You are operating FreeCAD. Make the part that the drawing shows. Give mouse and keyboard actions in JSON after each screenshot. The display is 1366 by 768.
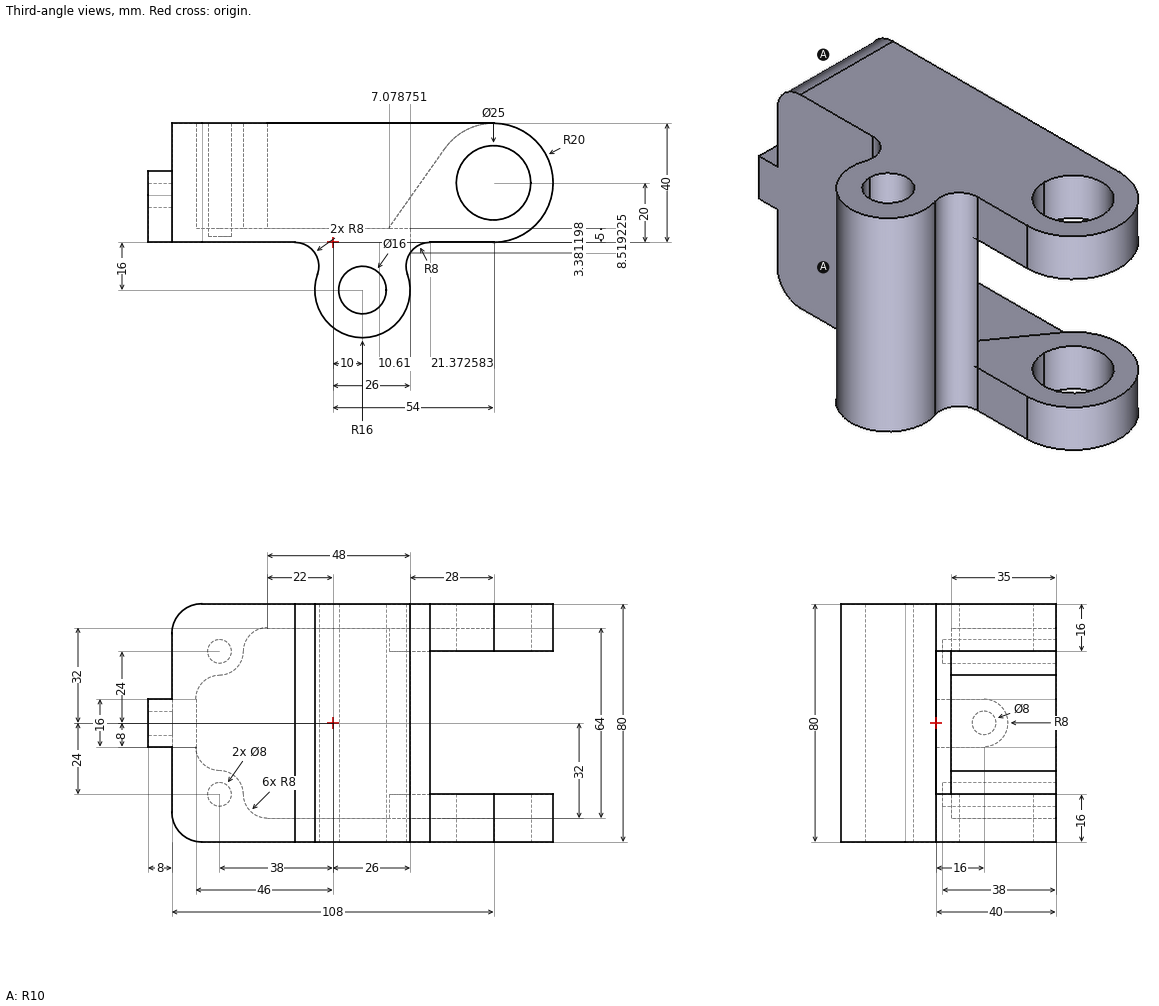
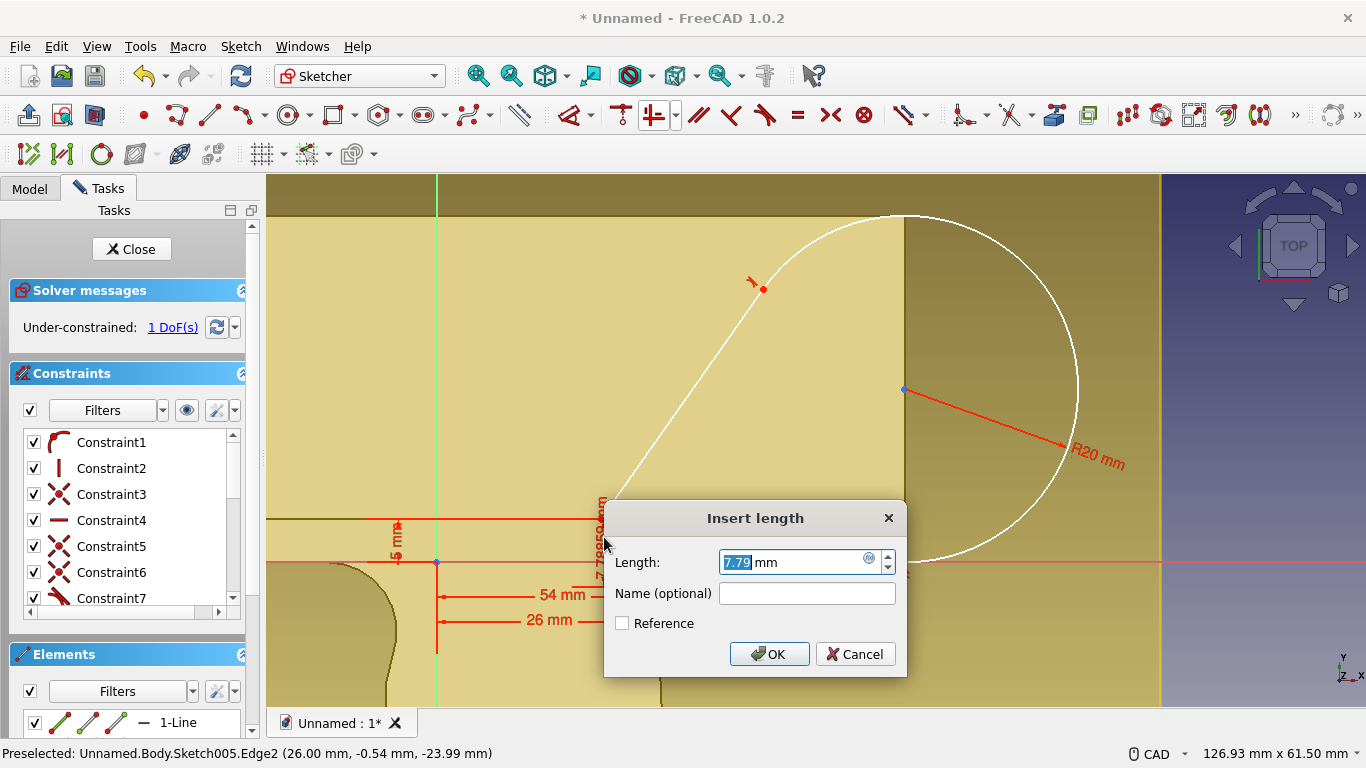
{"action": "type", "text": "8.519225"}
{"action": "key", "text": "Return"}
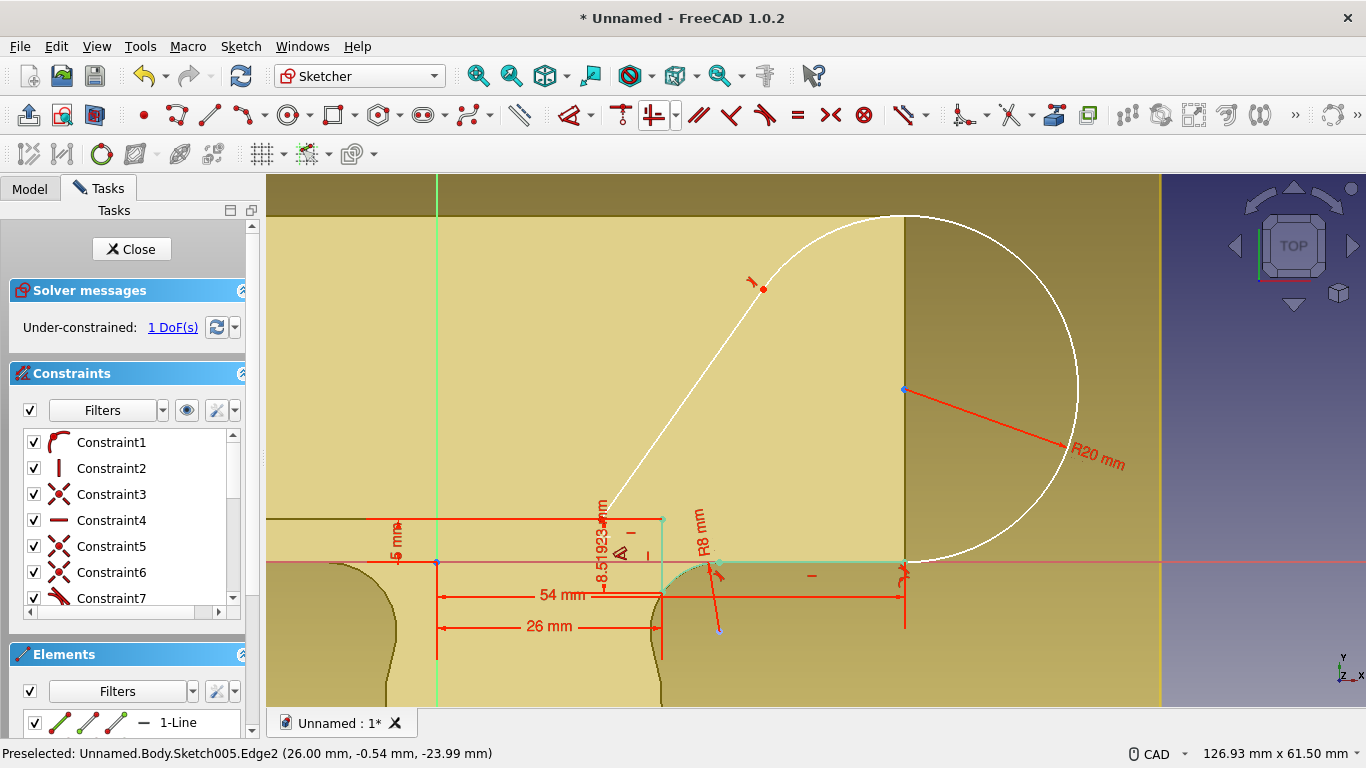
{"action": "left_click", "coordinate": [644, 519]}
{"action": "left_click", "coordinate": [646, 485]}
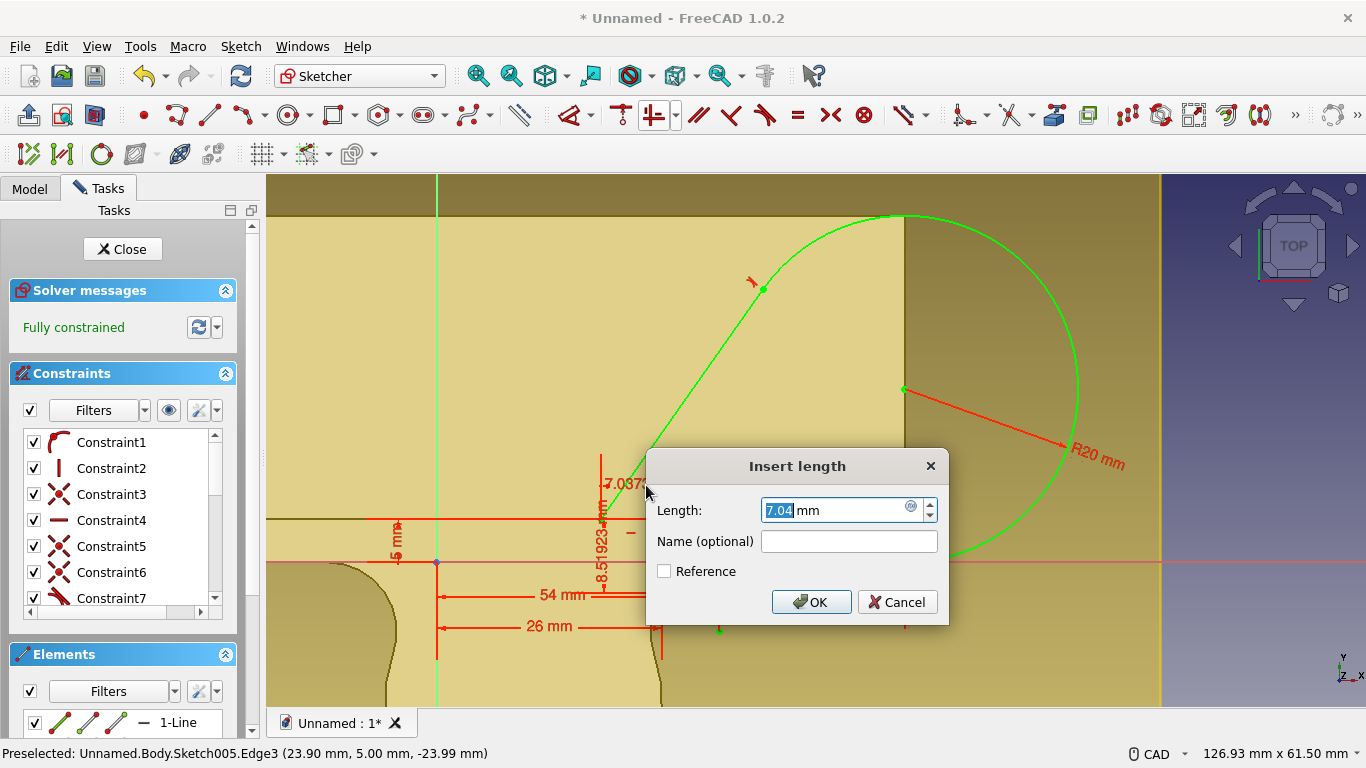
{"action": "type", "text": "7.078751"}
{"action": "key", "text": "Return"}
{"action": "key", "text": "Escape"}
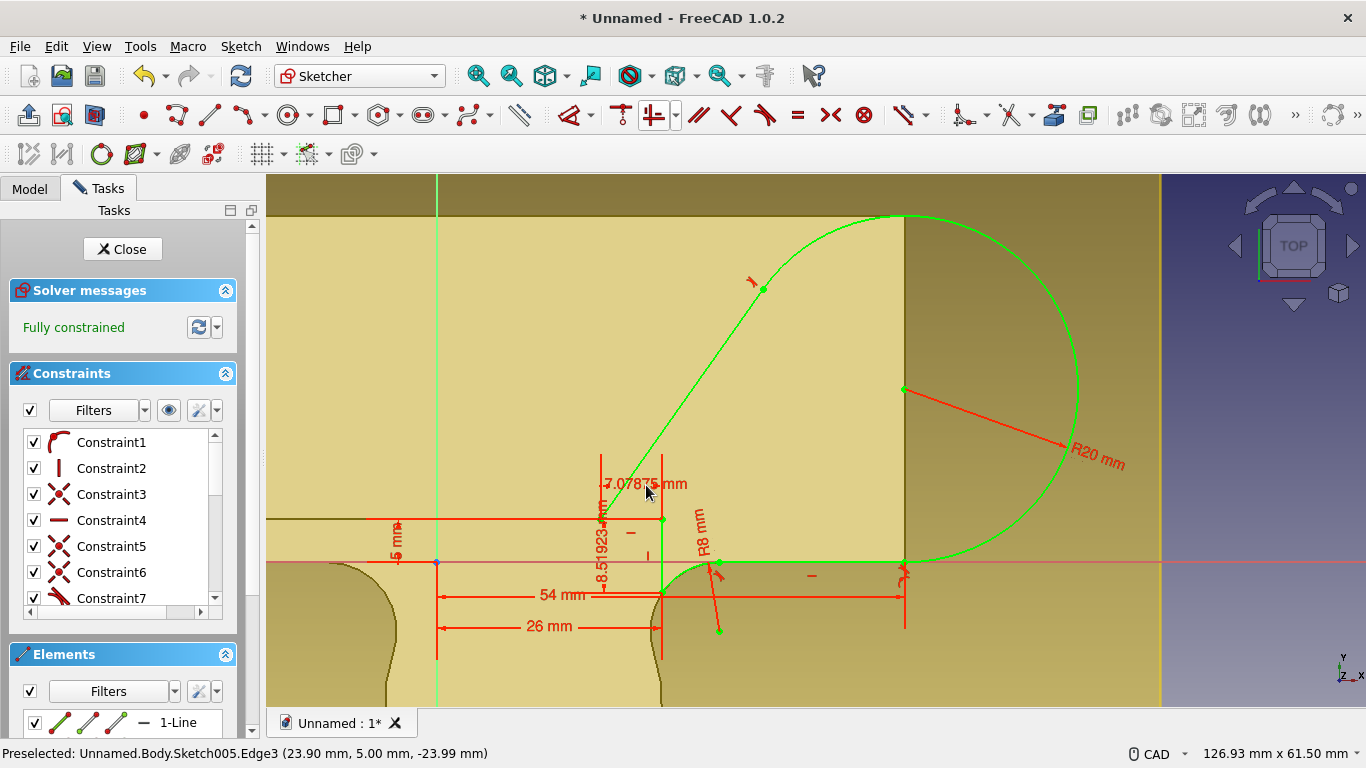
{"action": "left_click", "coordinate": [123, 249]}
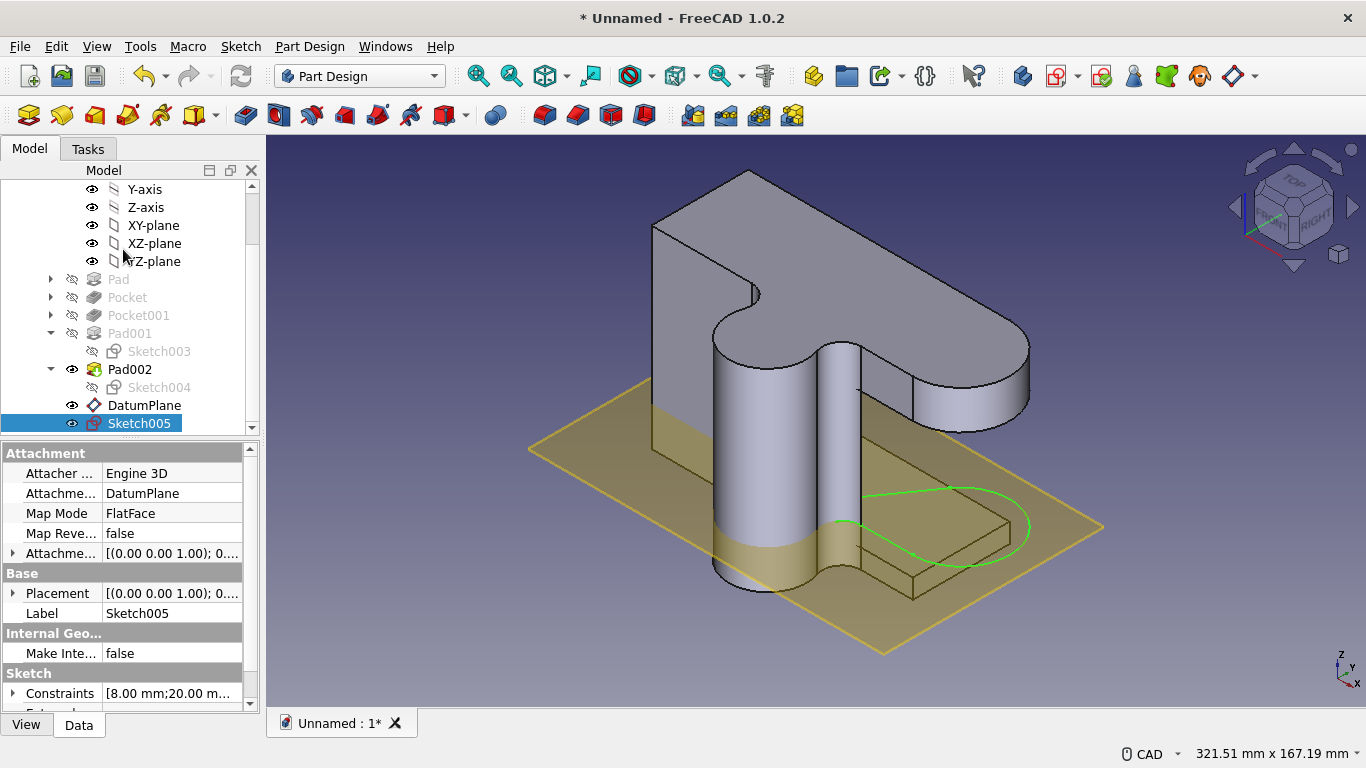
{"action": "left_click", "coordinate": [29, 116]}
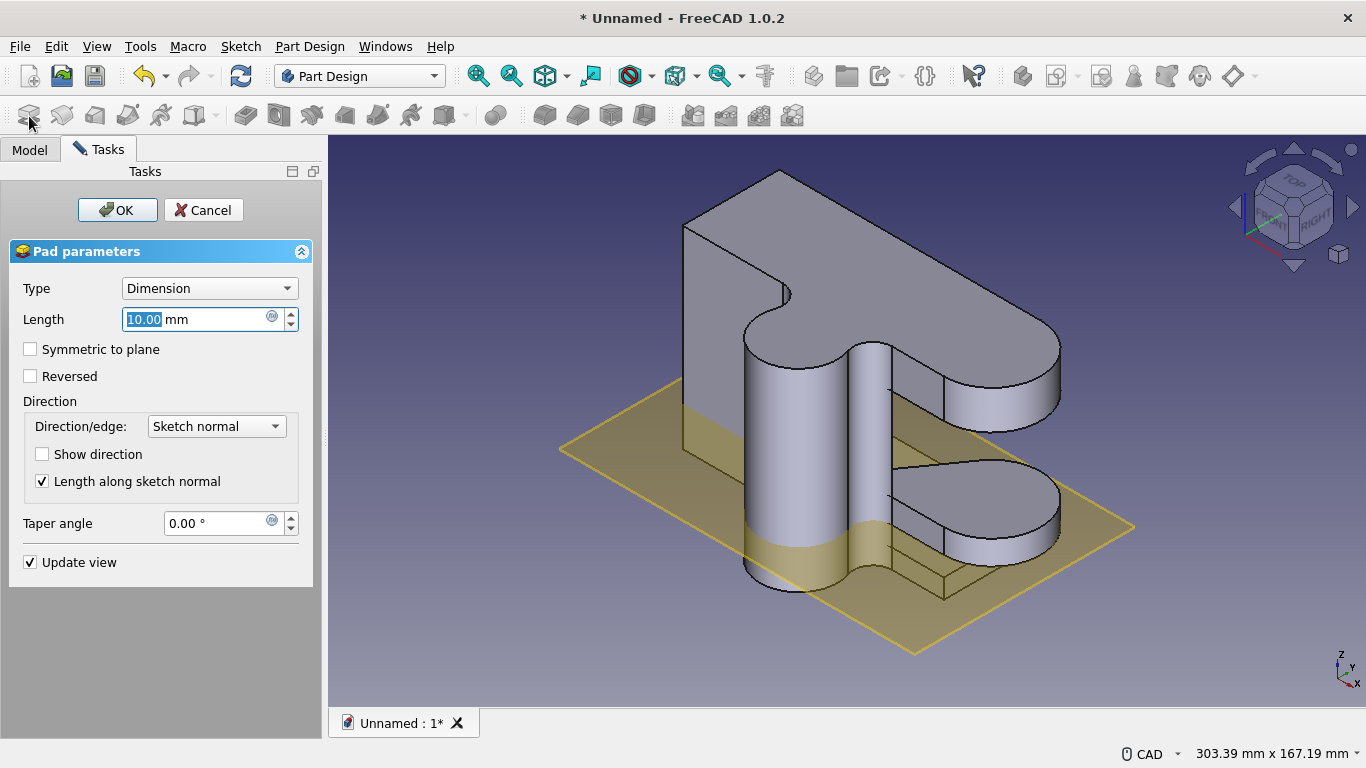
{"action": "type", "text": "16"}
{"action": "key", "text": "Tab"}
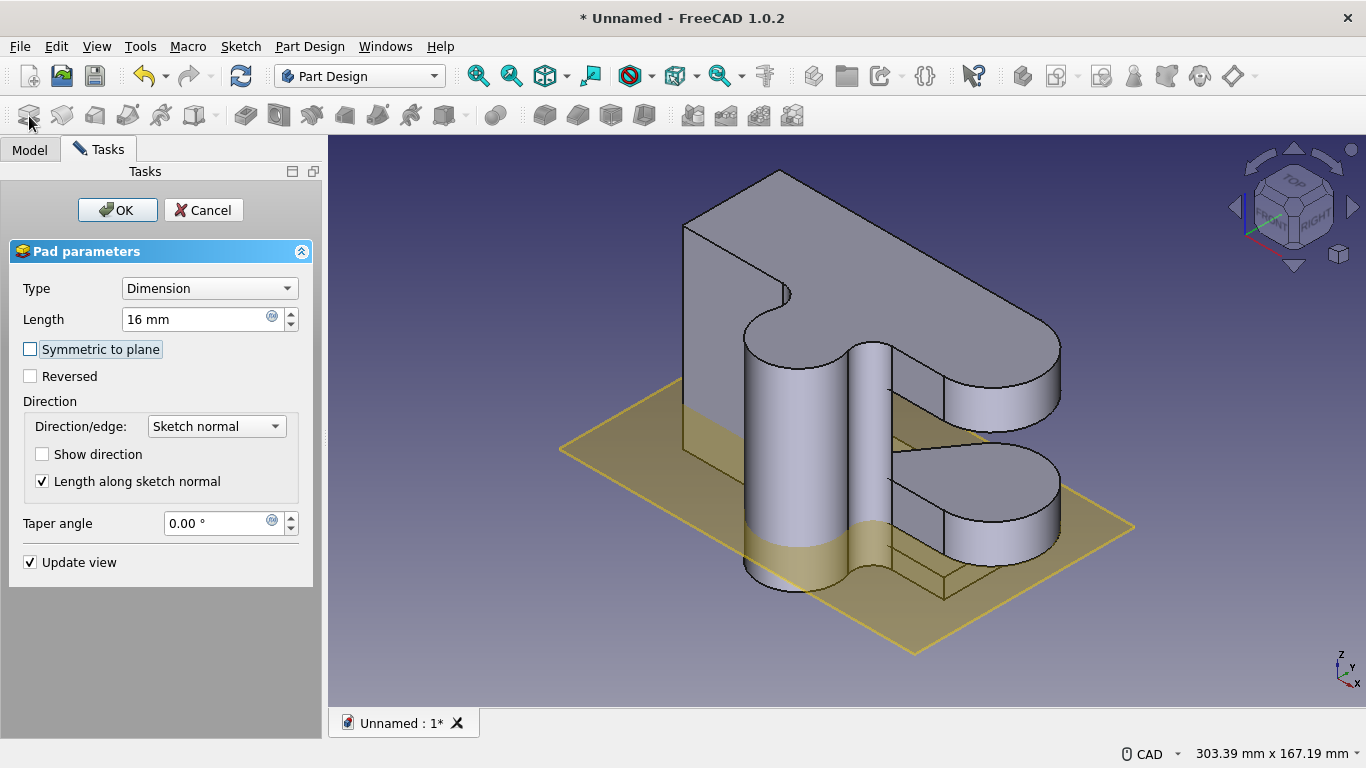
{"action": "left_click", "coordinate": [31, 376]}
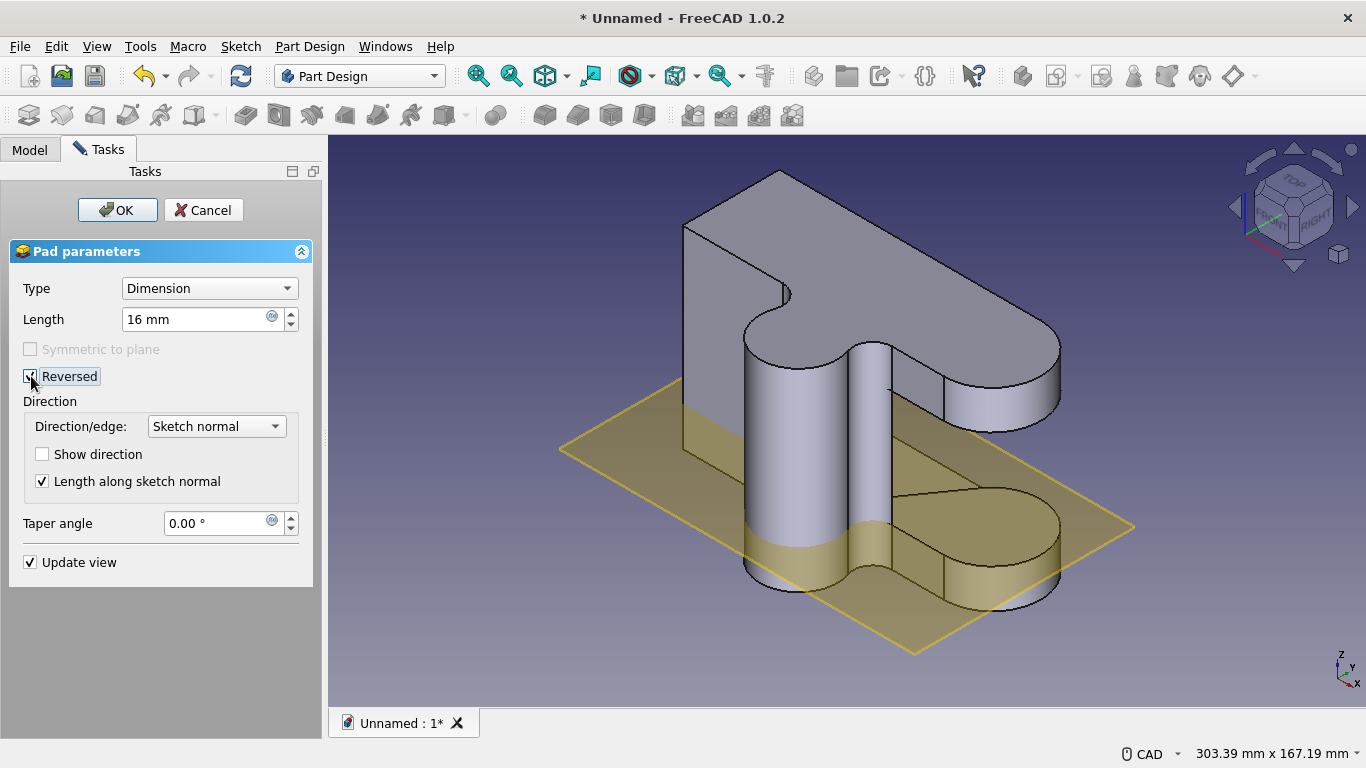
{"action": "left_click", "coordinate": [118, 210]}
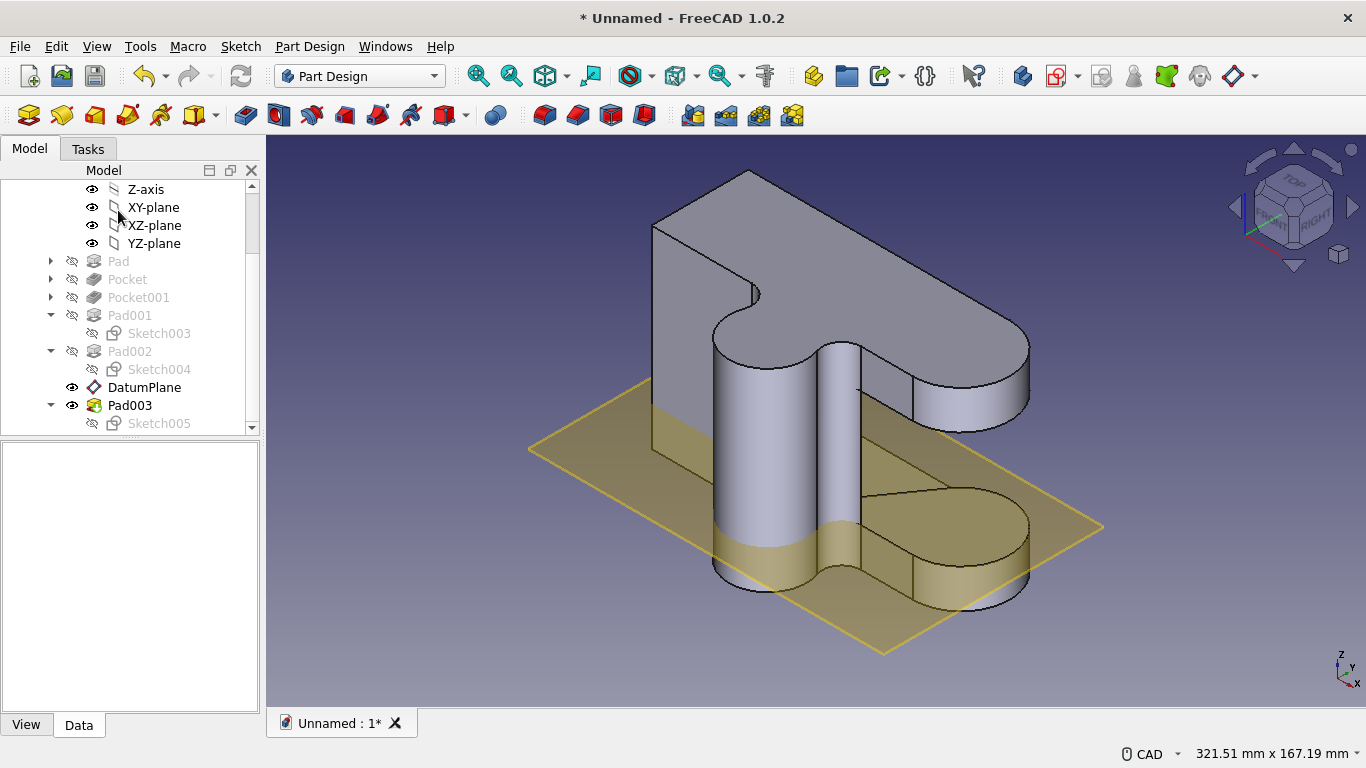
{"action": "left_click", "coordinate": [117, 387]}
{"action": "key", "text": "space"}